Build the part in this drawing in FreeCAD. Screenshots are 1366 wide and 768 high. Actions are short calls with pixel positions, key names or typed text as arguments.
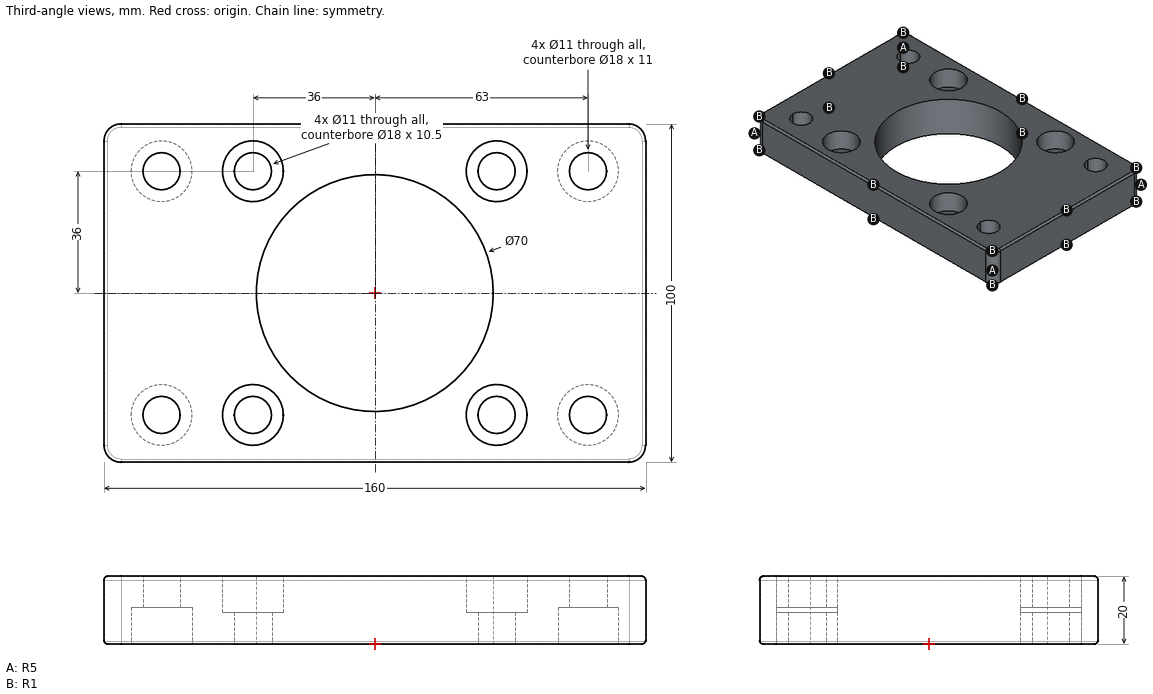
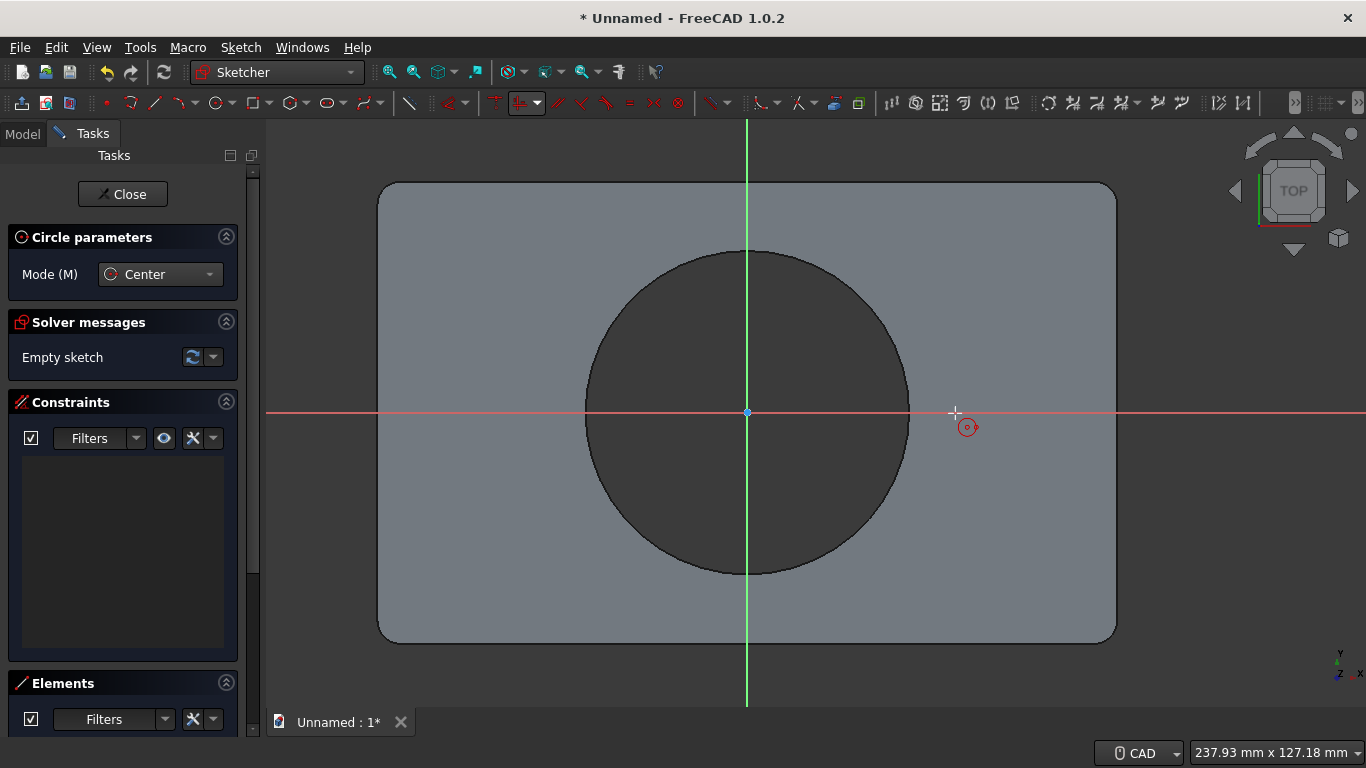
click(581, 246)
click(599, 228)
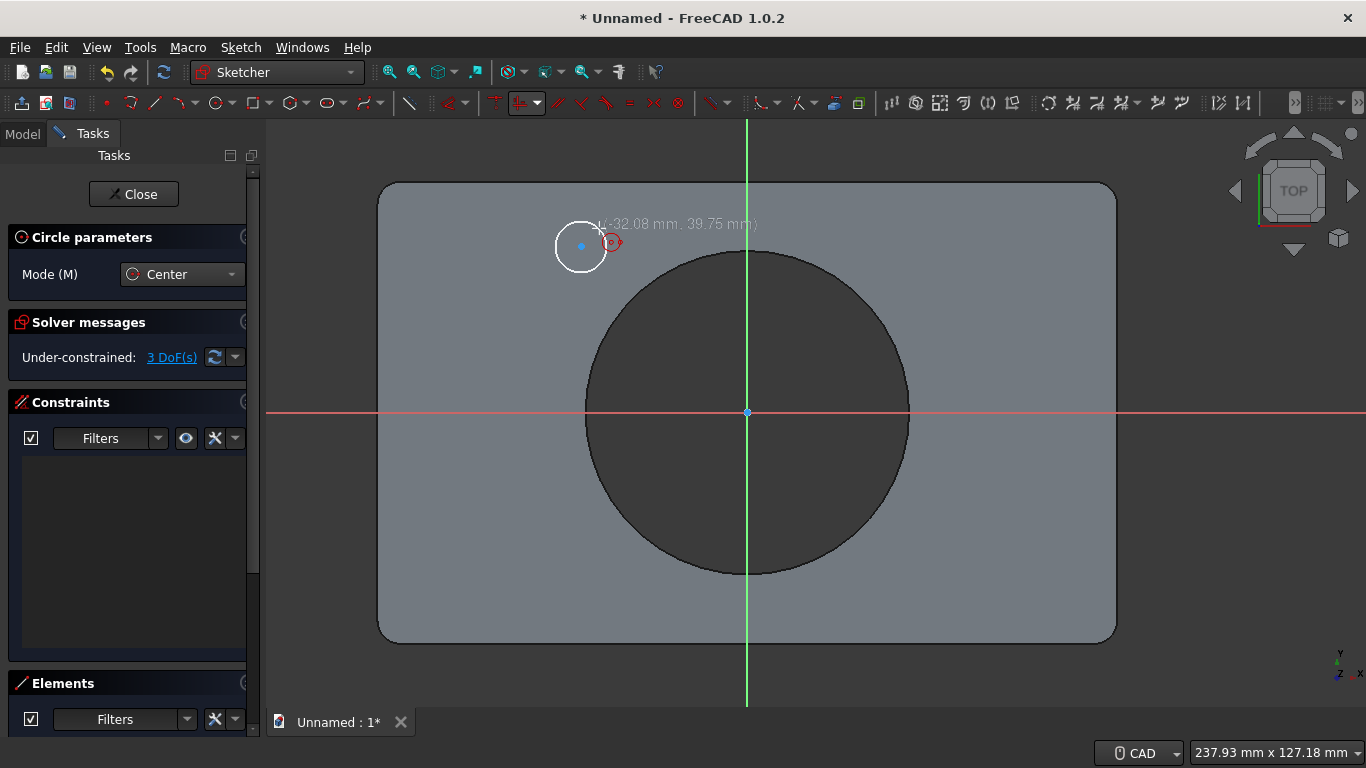
click(914, 246)
click(932, 228)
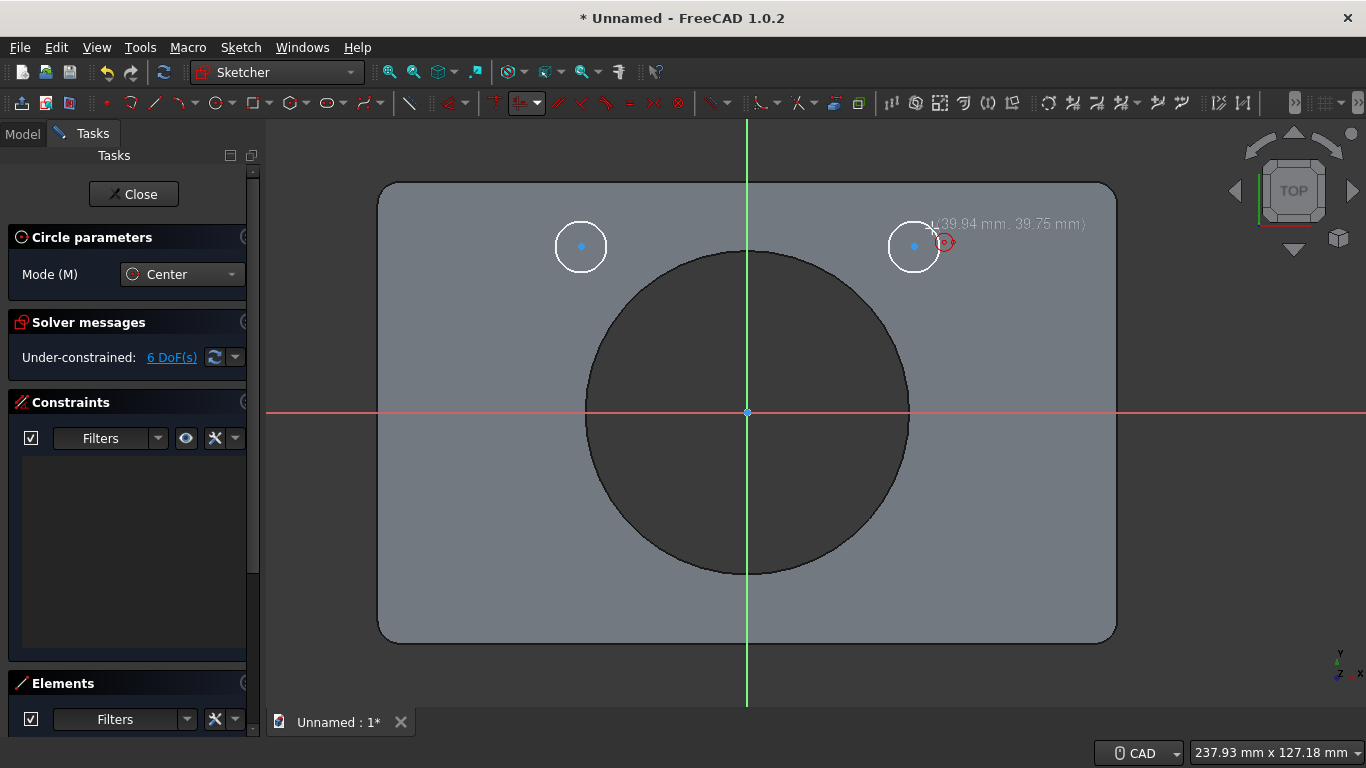
click(581, 579)
click(599, 561)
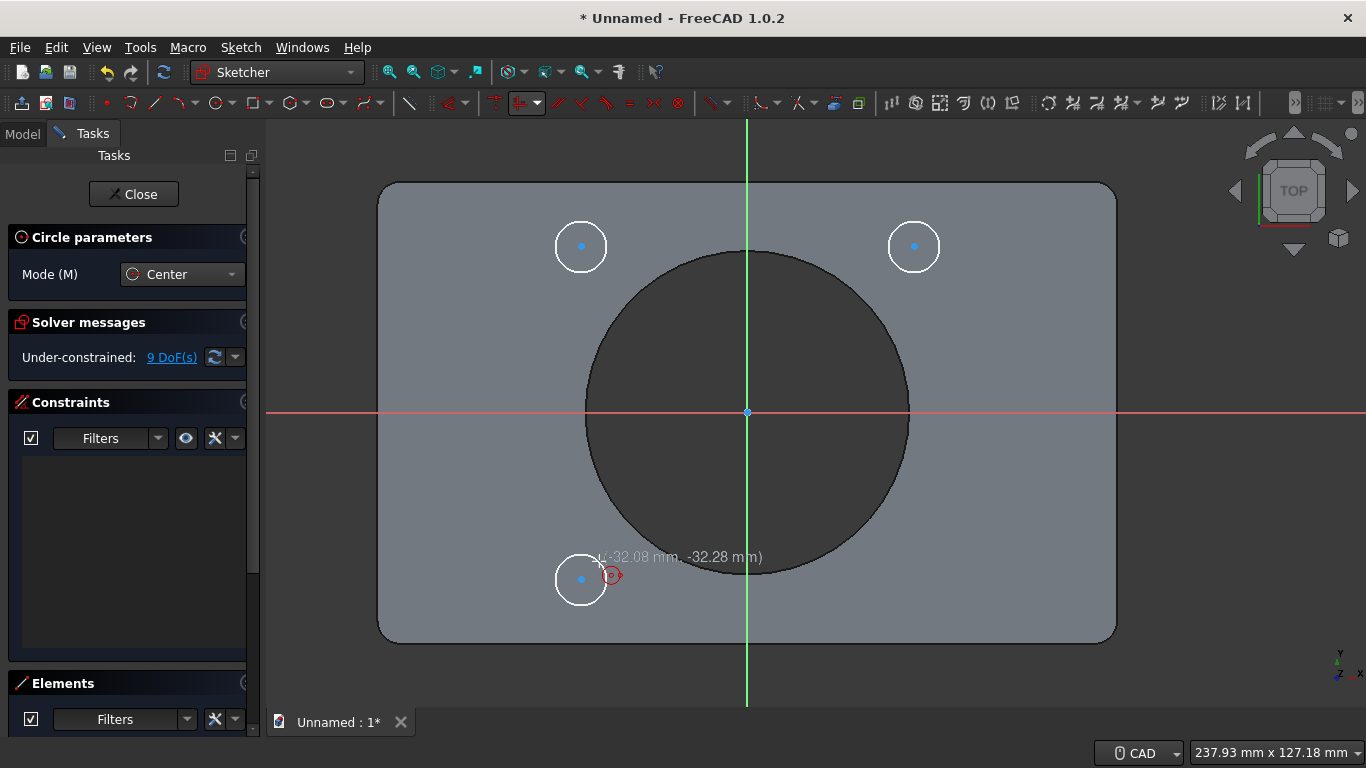
click(914, 579)
click(932, 561)
key(Escape)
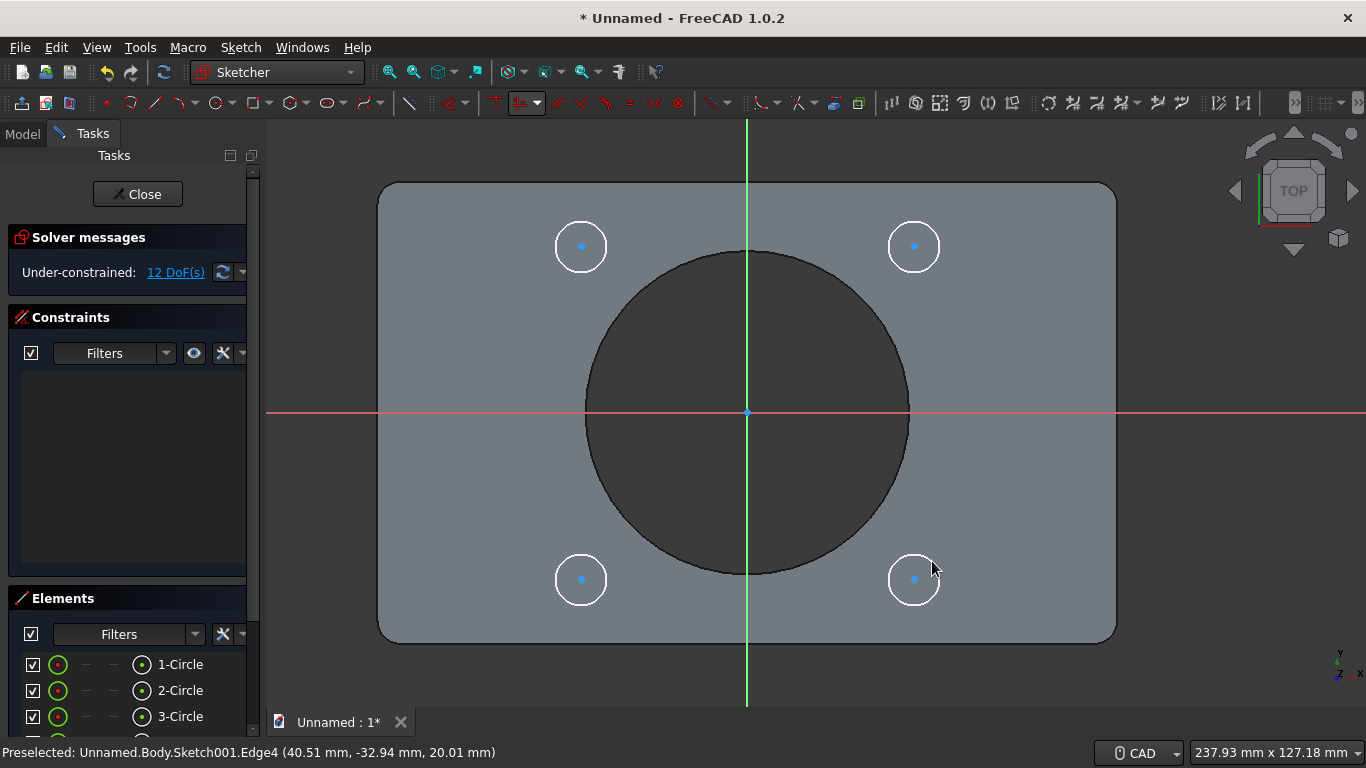
click(599, 229)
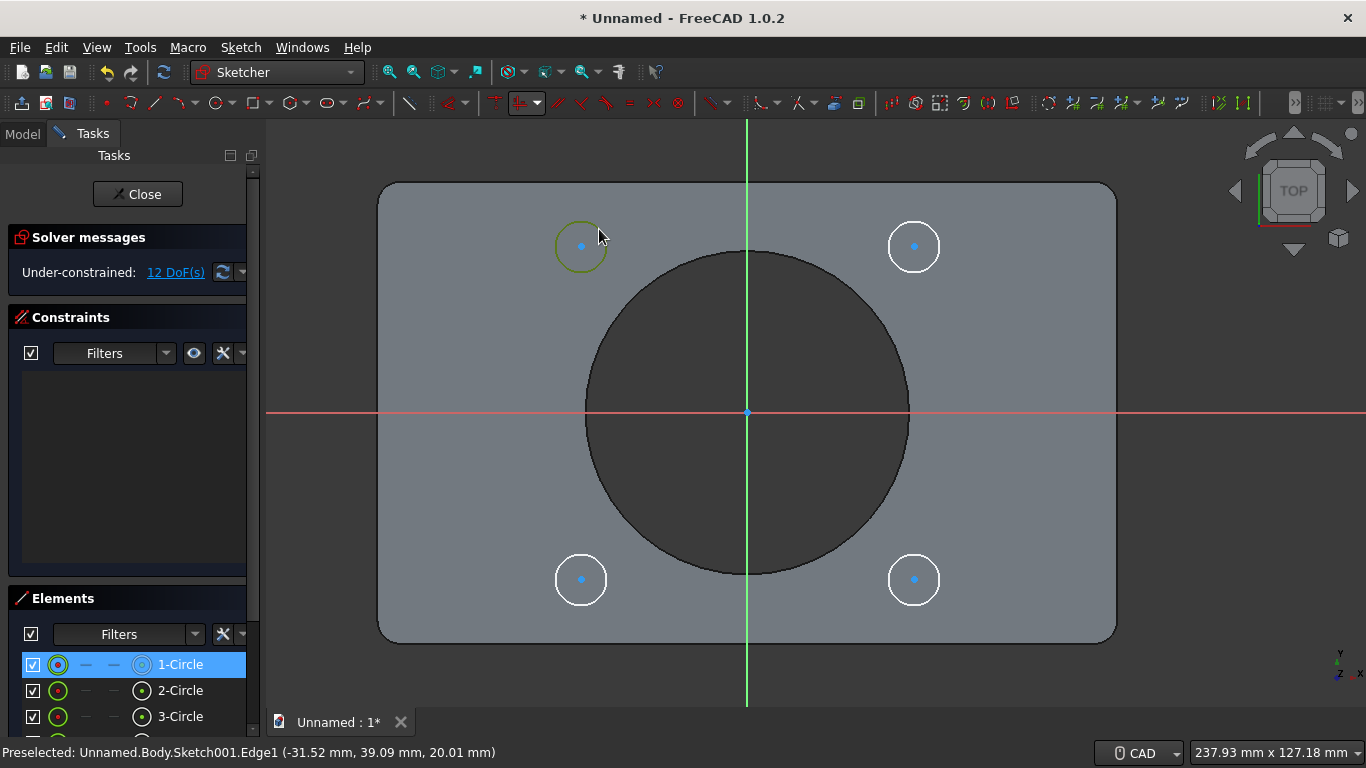
click(932, 229)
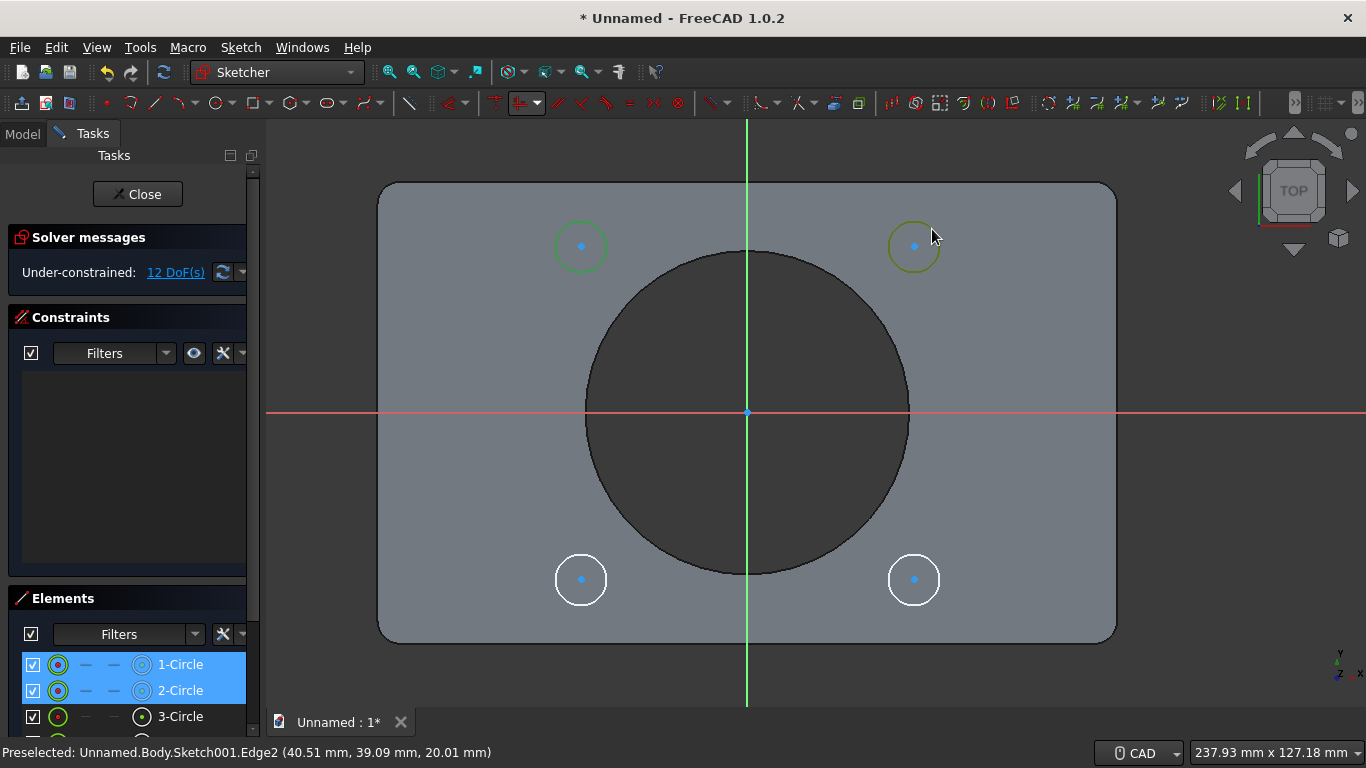
click(599, 562)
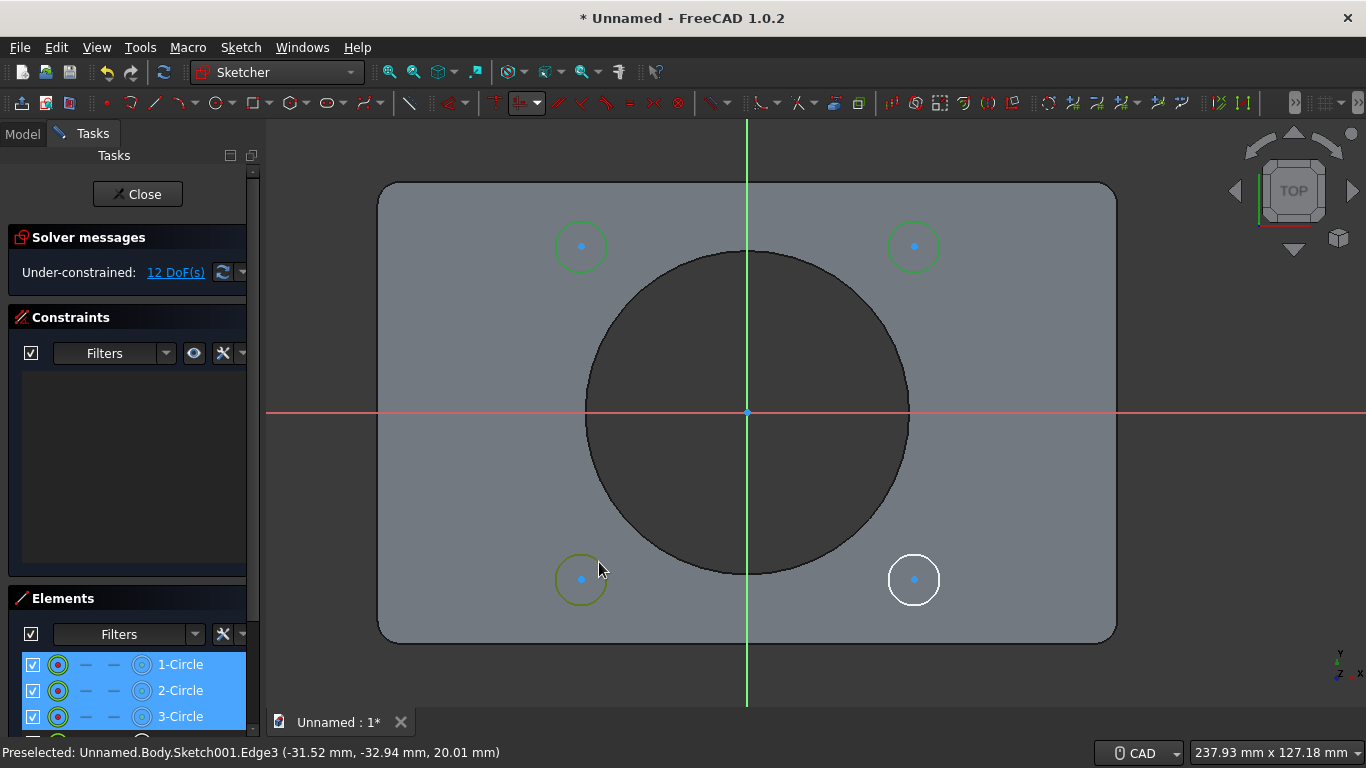
click(932, 562)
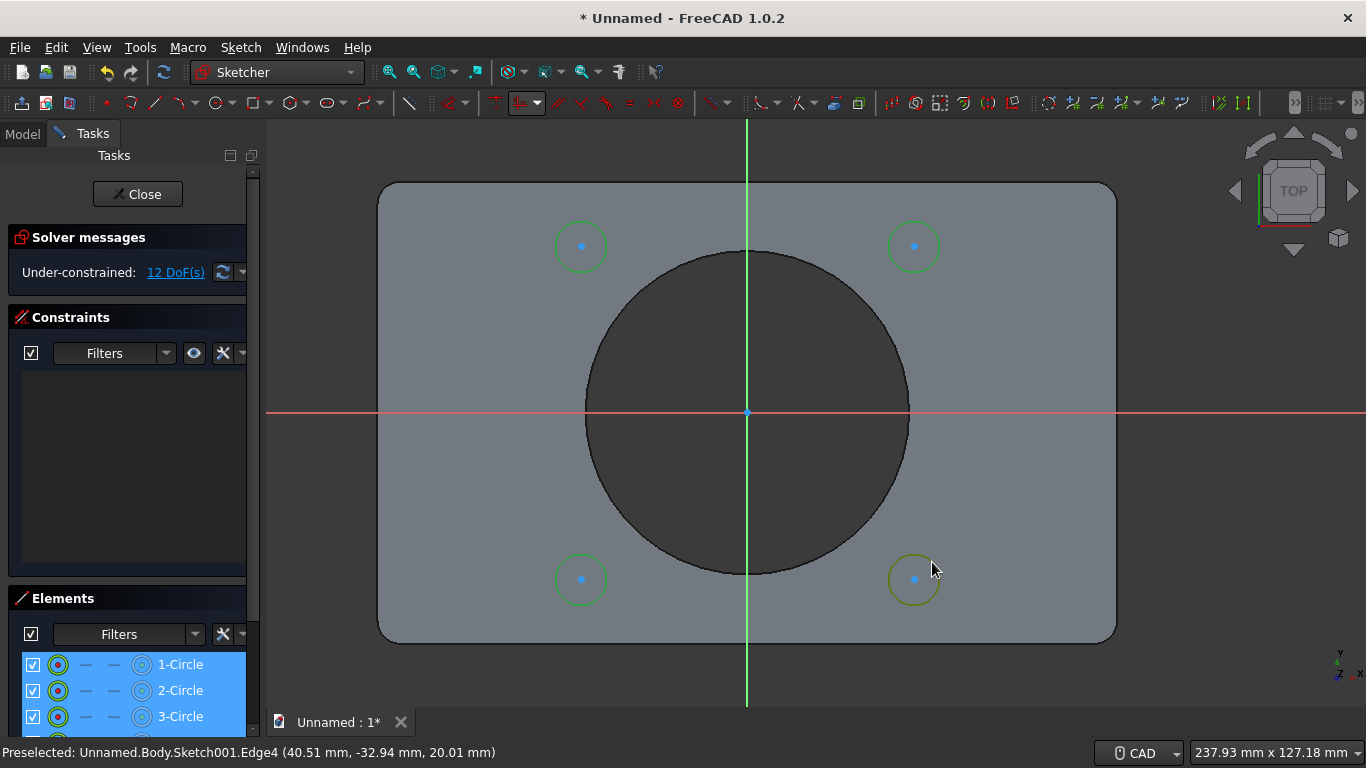
key(e)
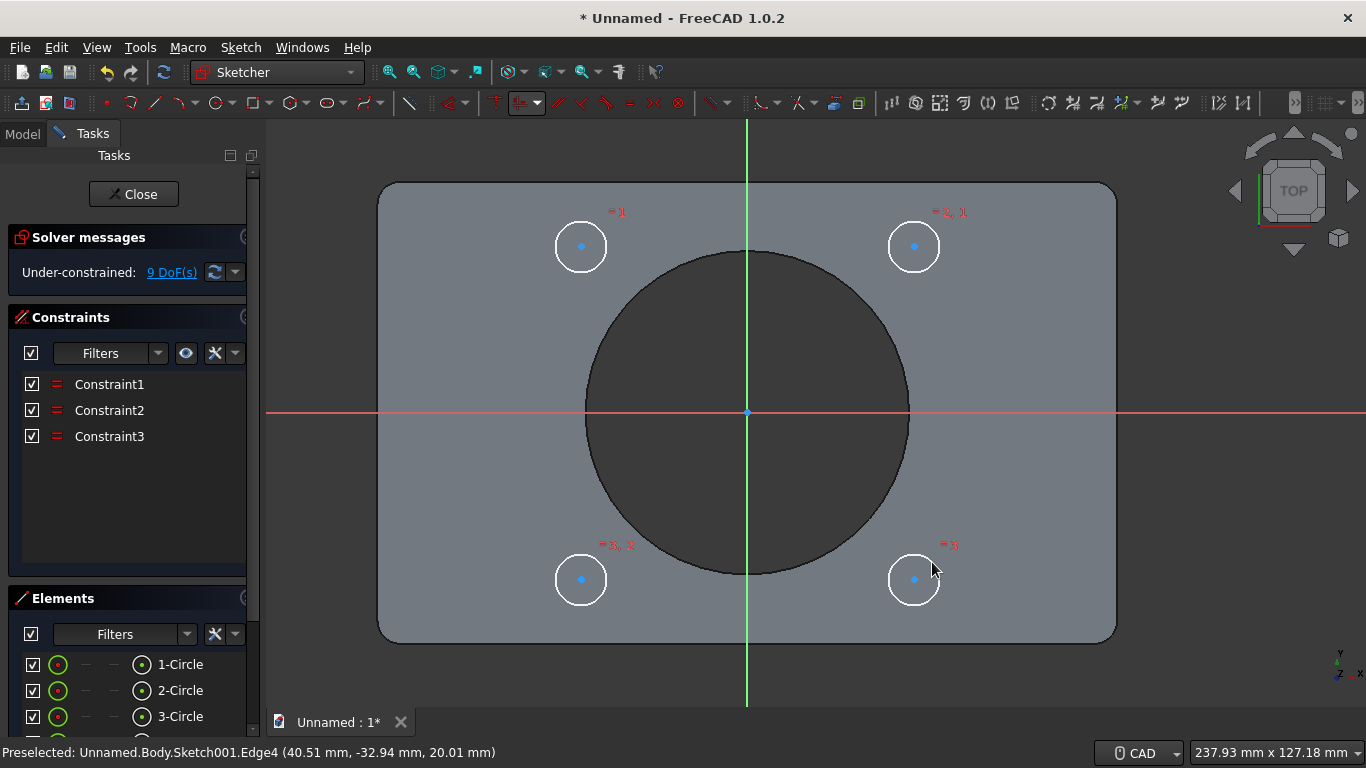
click(581, 247)